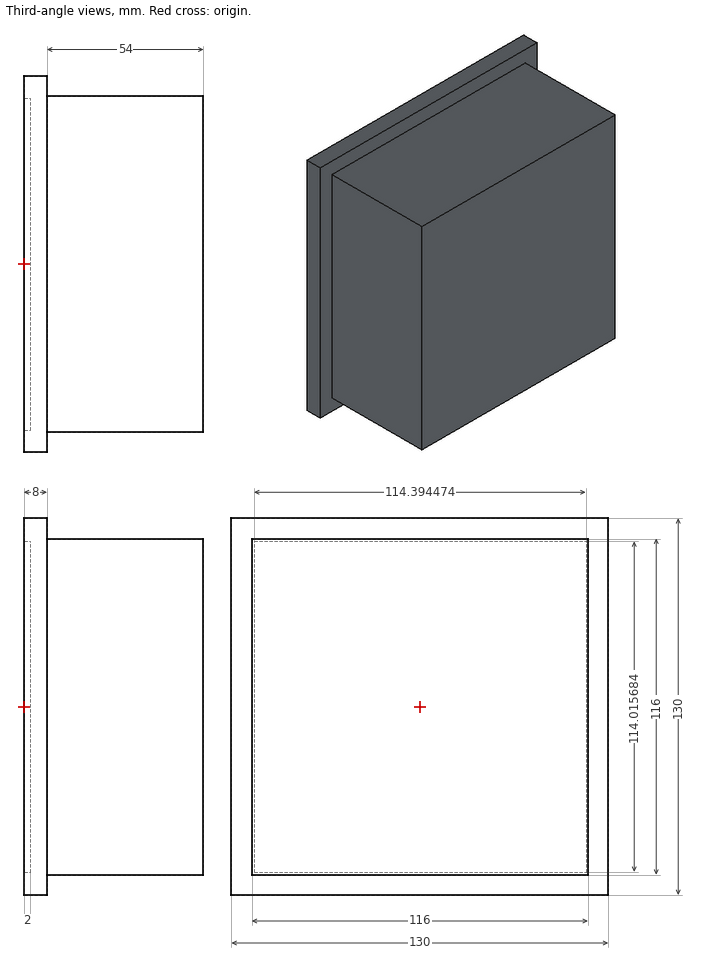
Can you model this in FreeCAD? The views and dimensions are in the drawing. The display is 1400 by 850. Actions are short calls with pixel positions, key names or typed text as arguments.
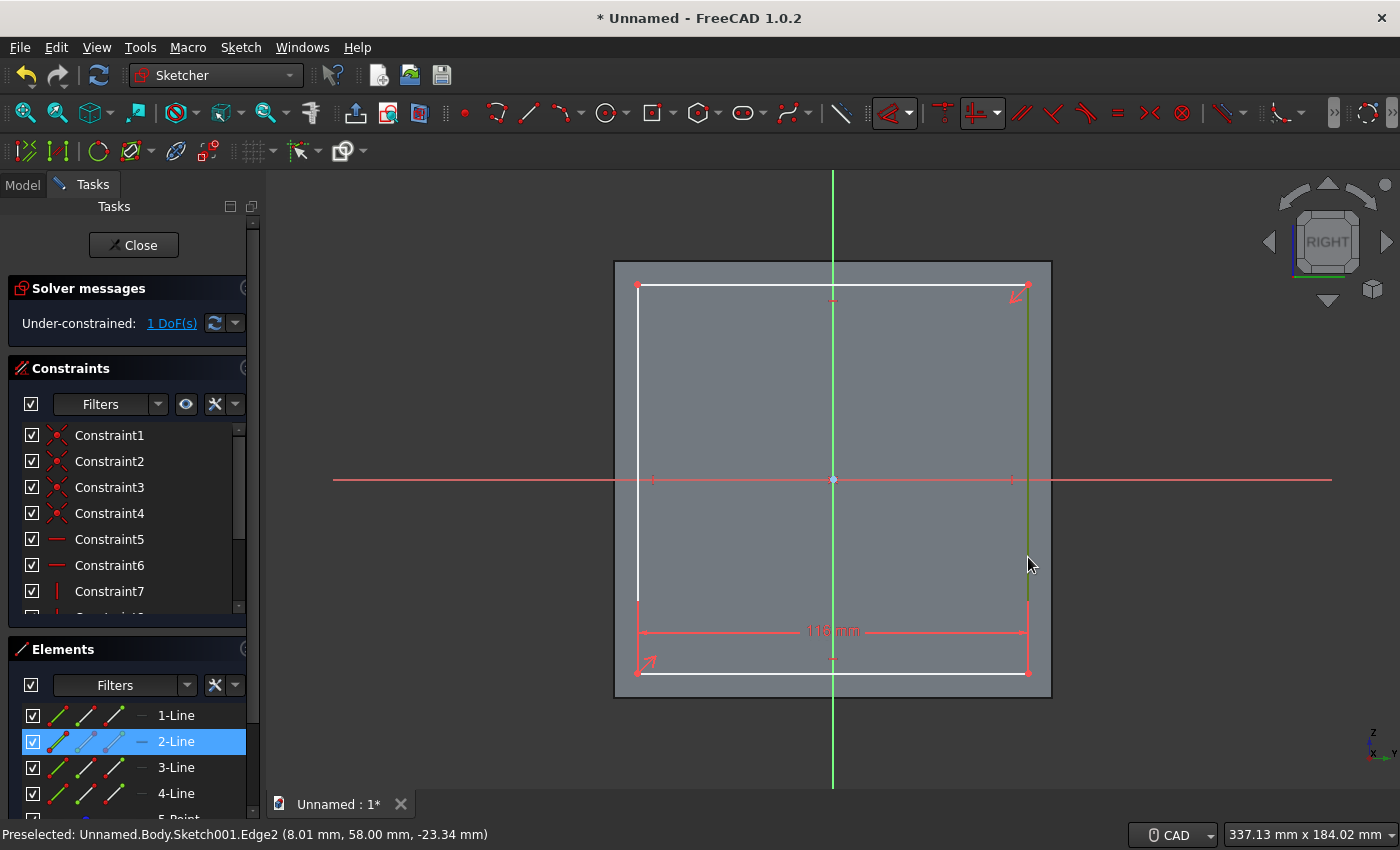
click(912, 114)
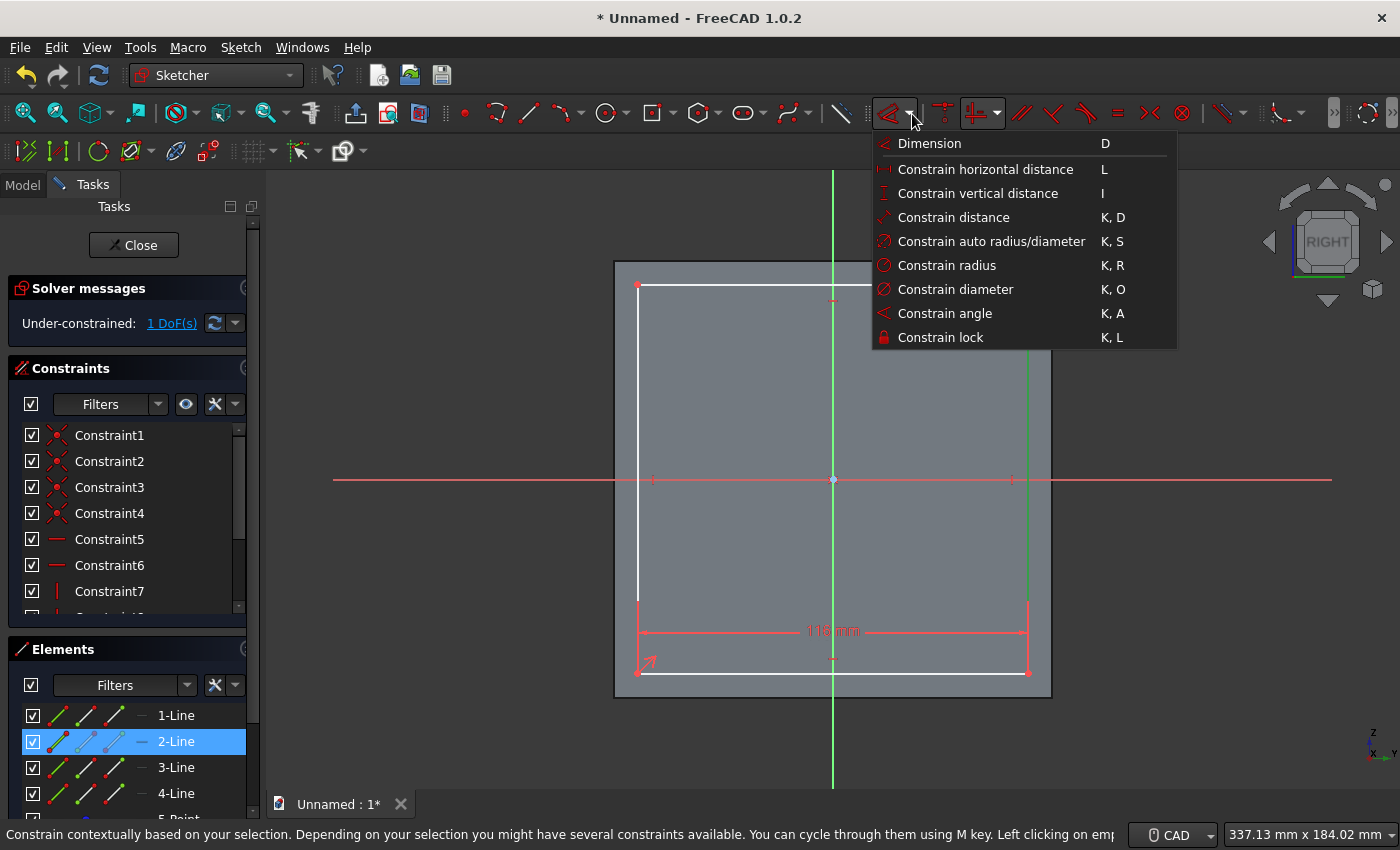
click(1025, 193)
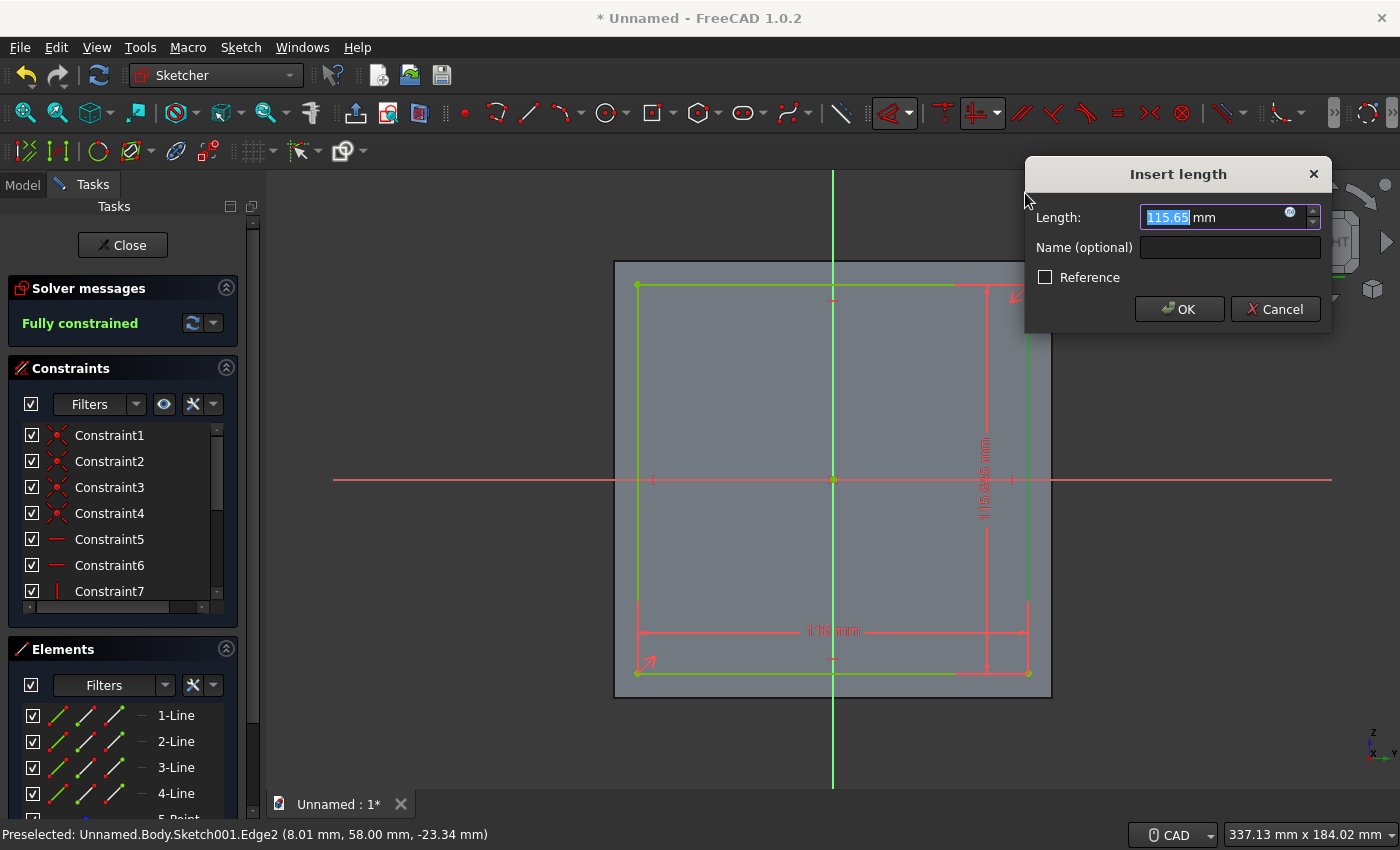
text(116)
key(Return)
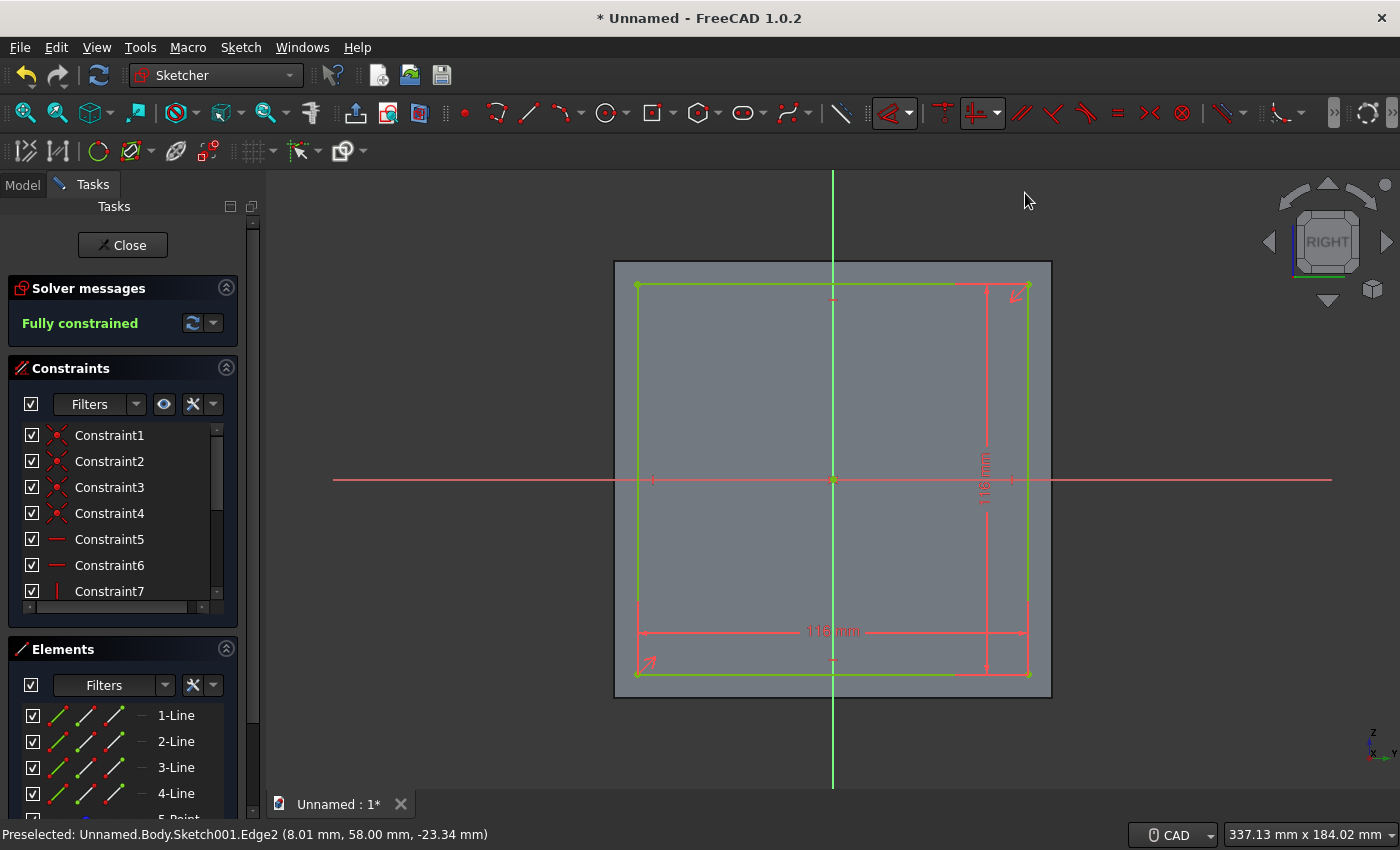
click(123, 245)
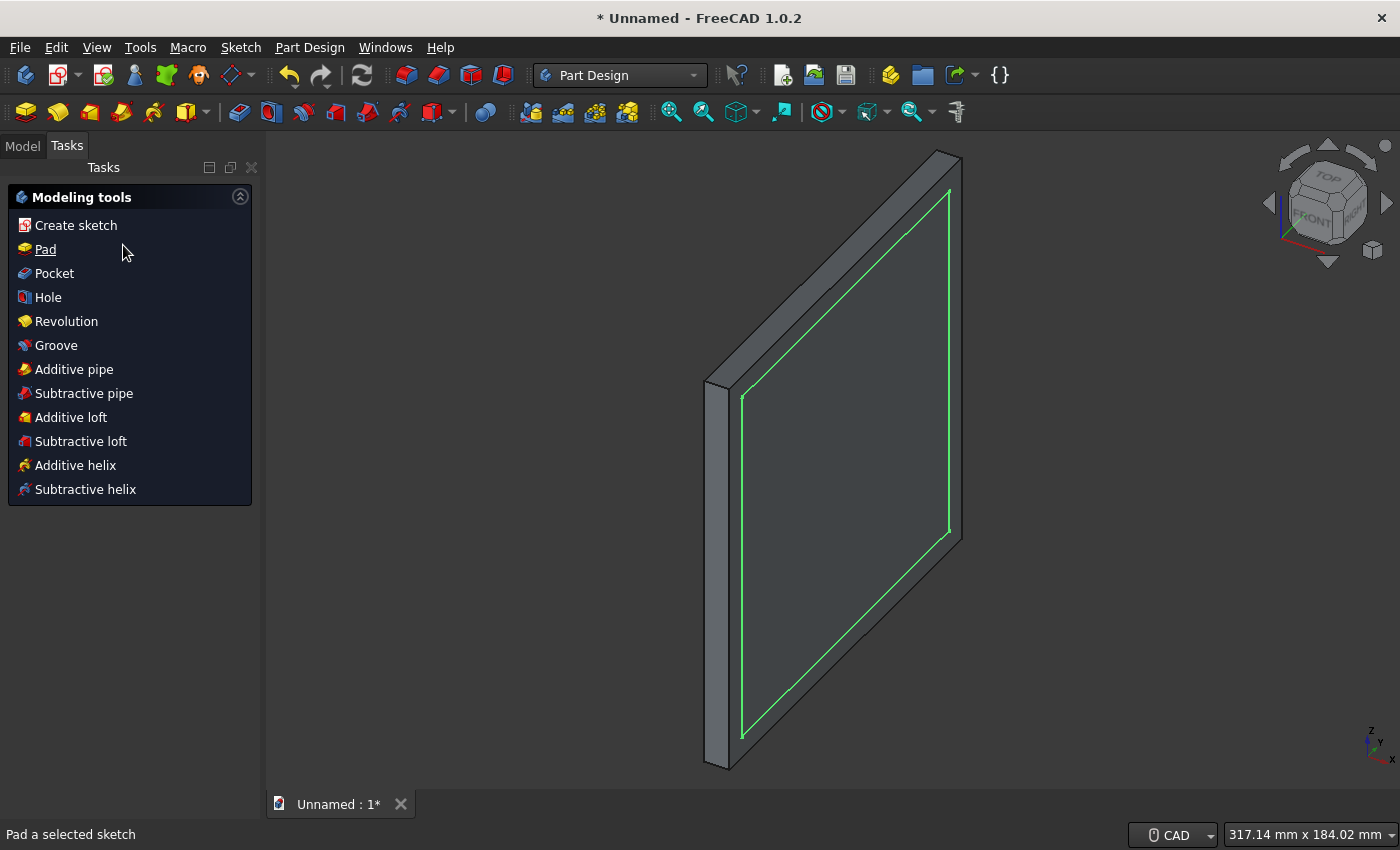
click(26, 112)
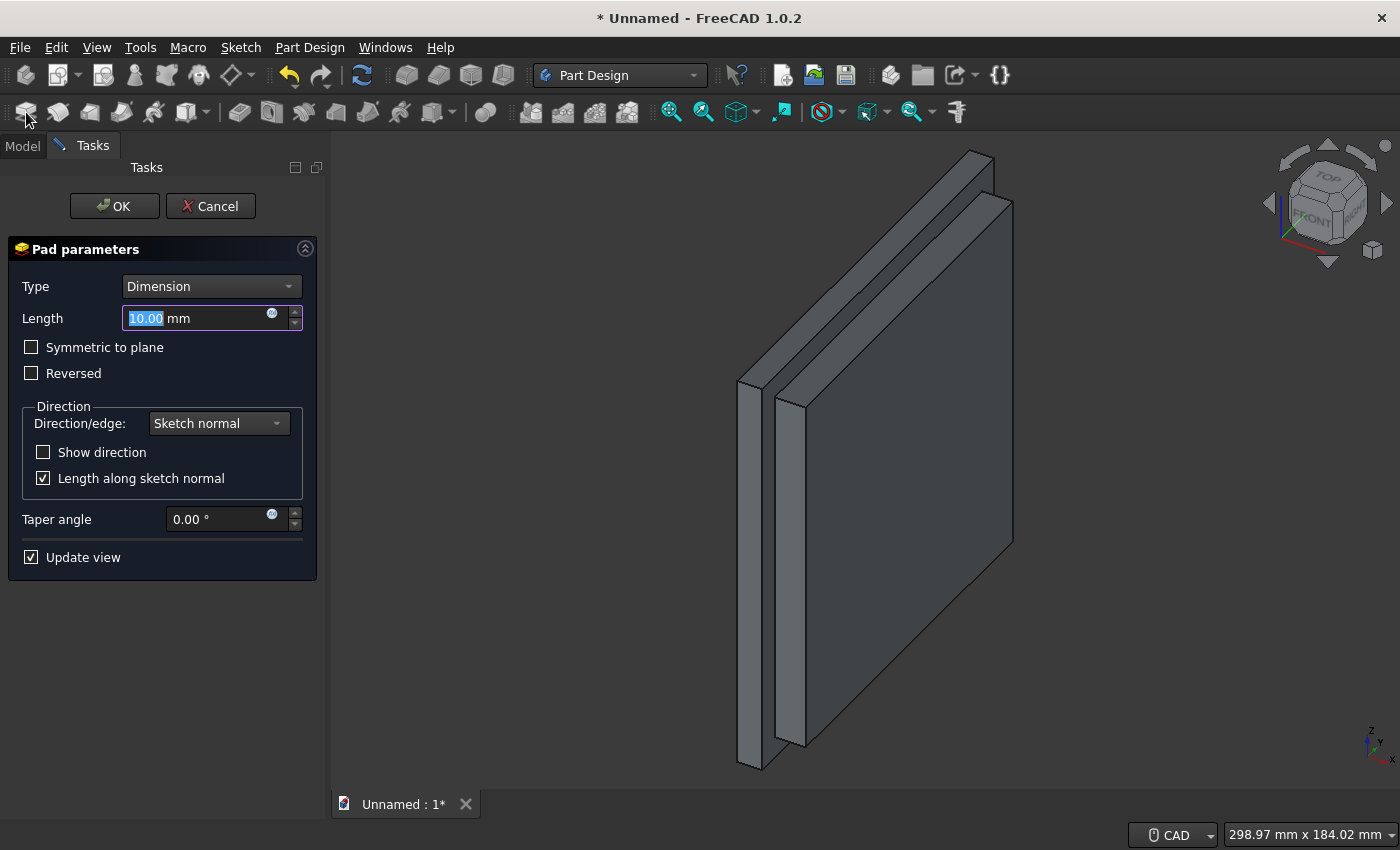
text(54)
key(Tab)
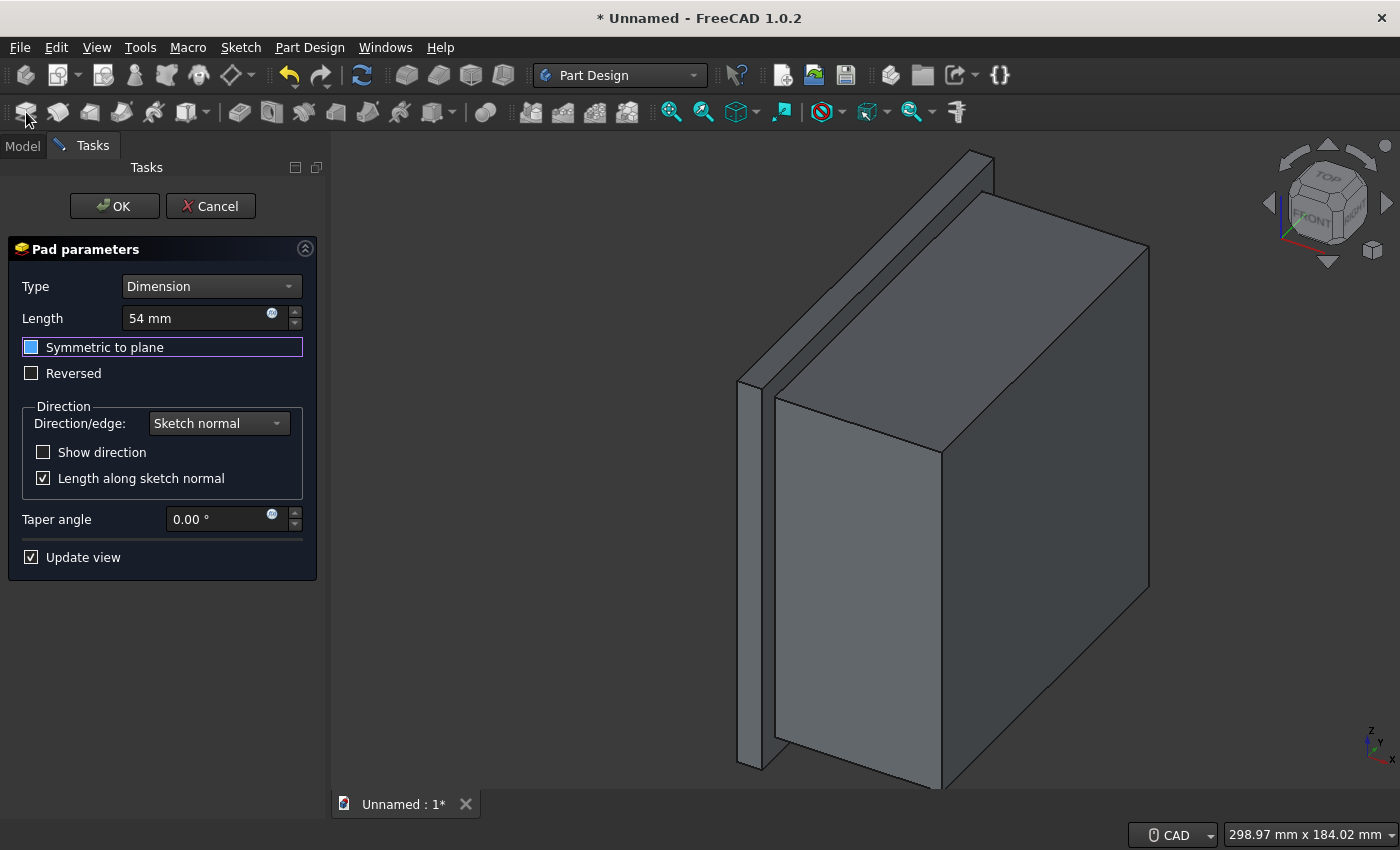
click(115, 206)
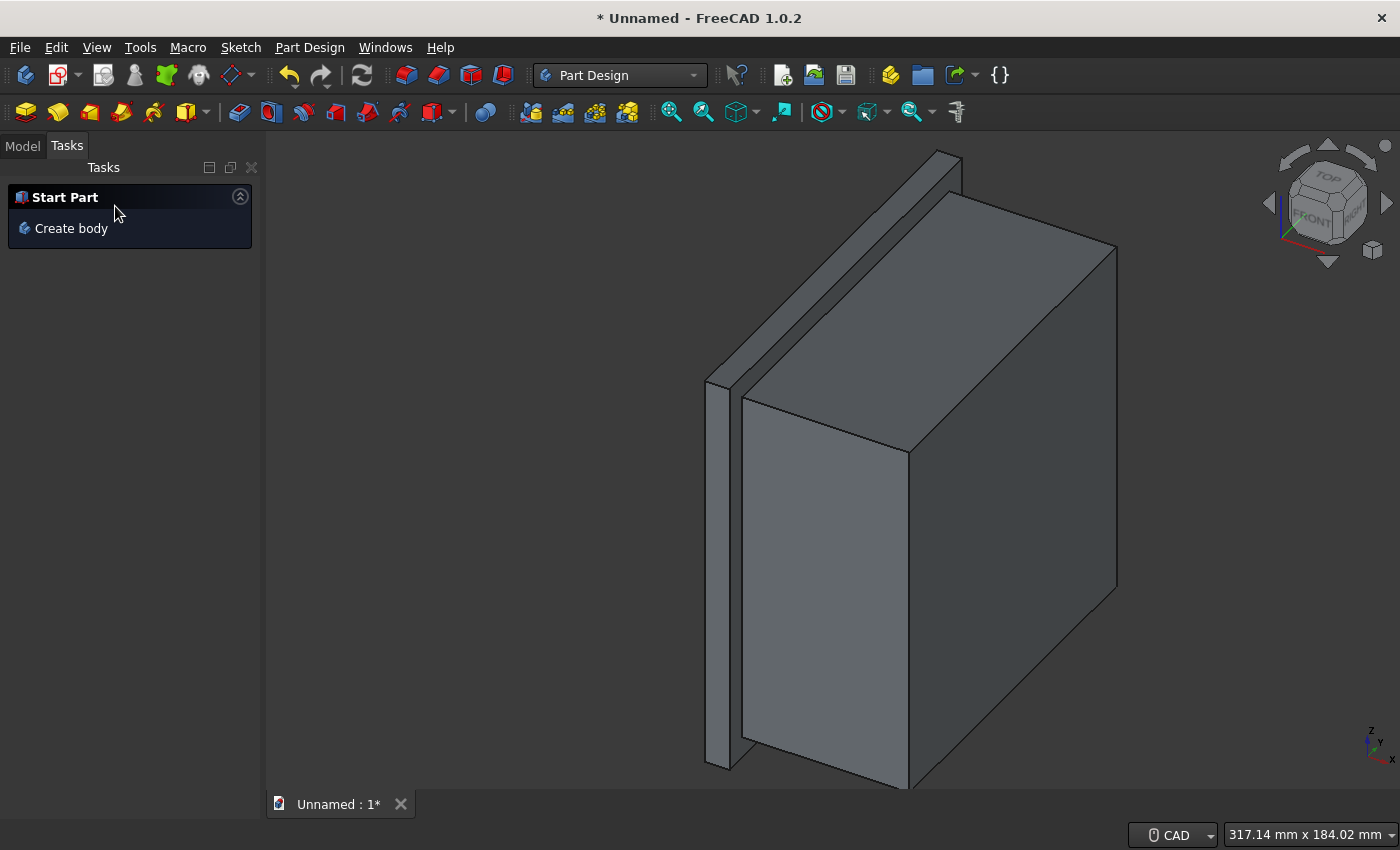
click(672, 112)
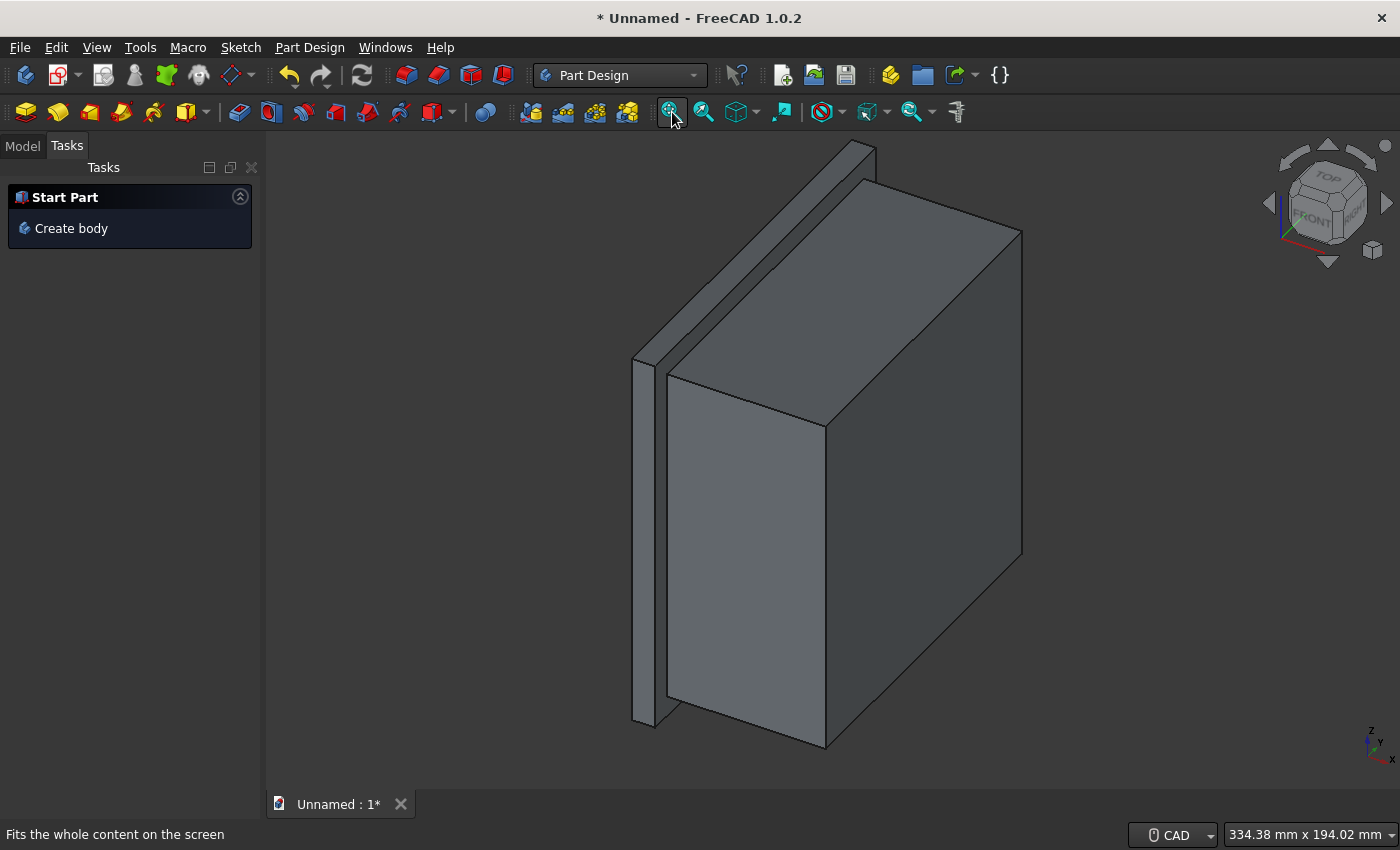
key(6)